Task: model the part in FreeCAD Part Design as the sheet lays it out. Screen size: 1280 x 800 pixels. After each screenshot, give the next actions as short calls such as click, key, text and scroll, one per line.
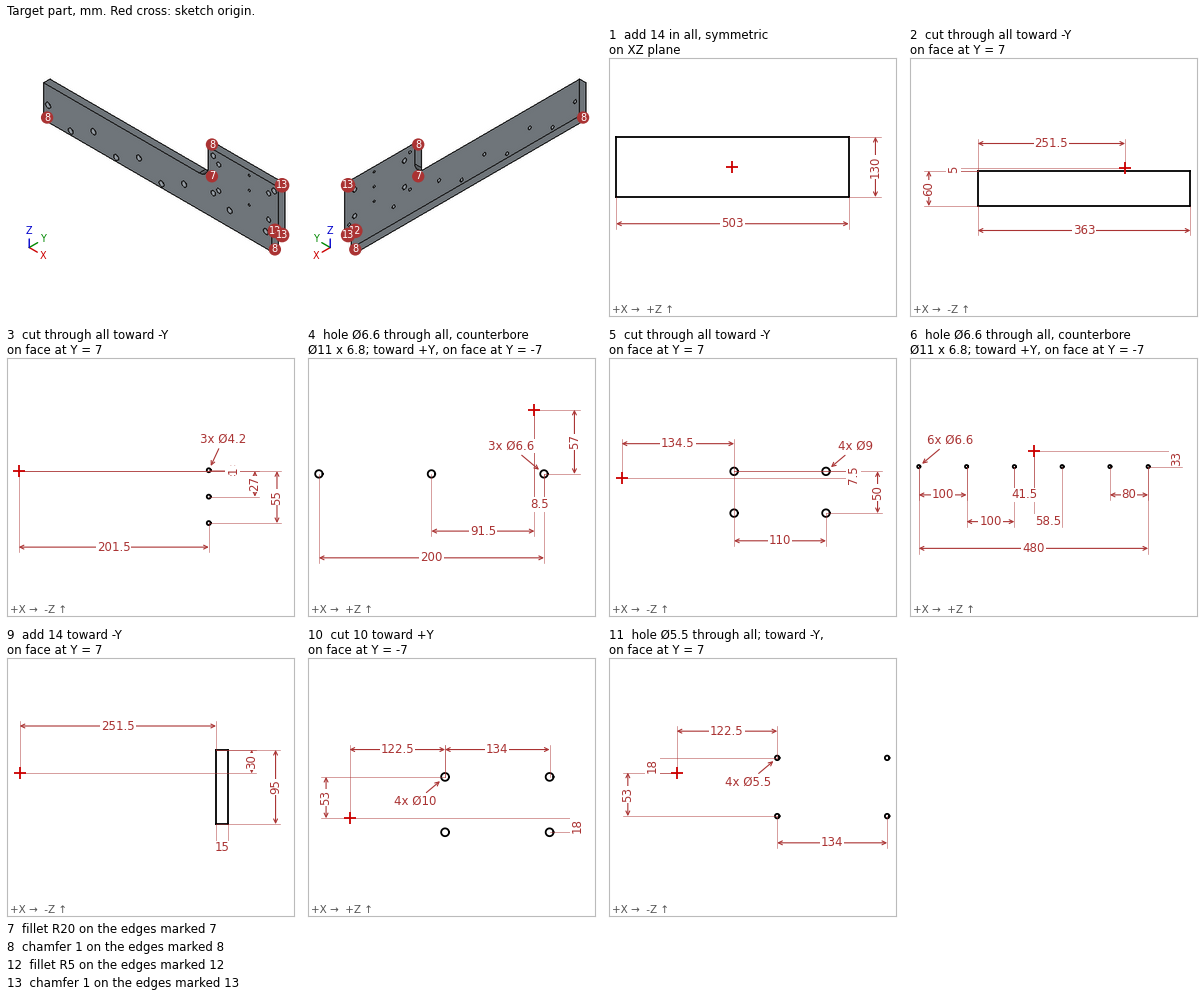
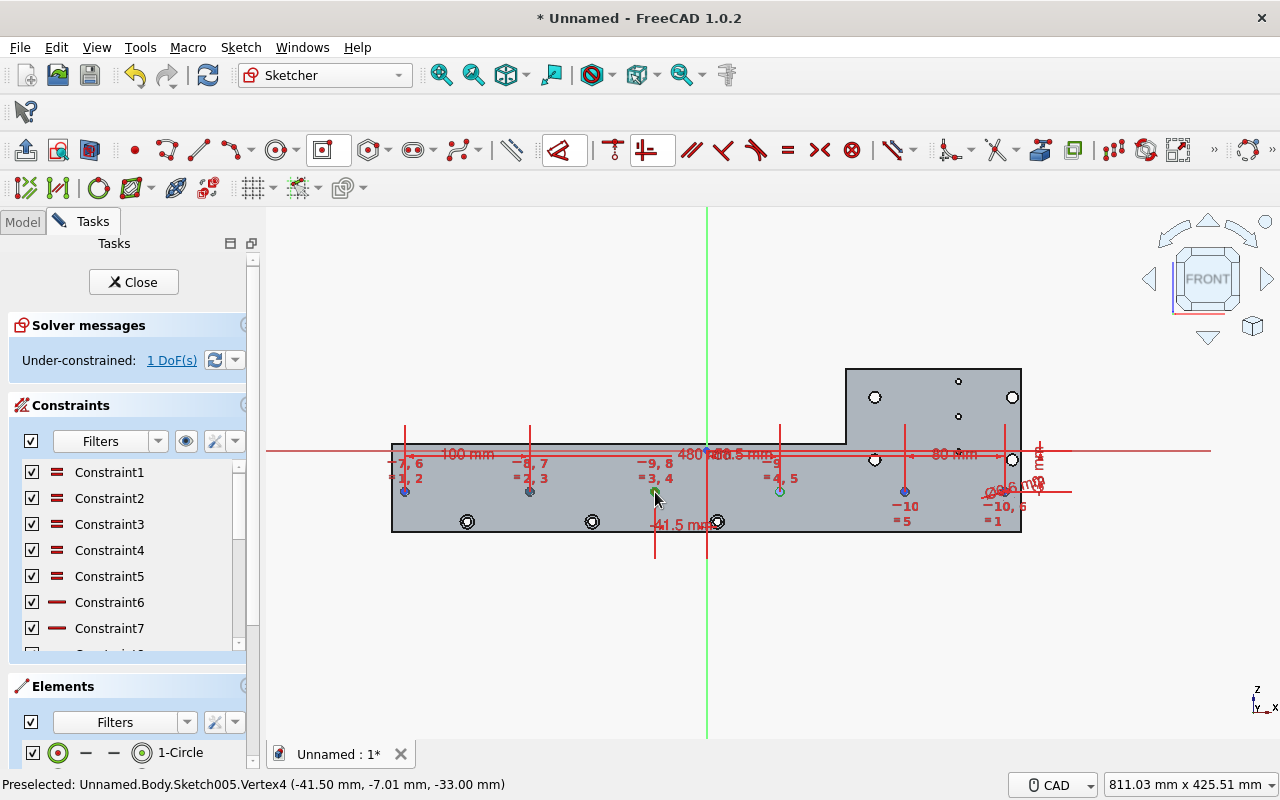
click(582, 150)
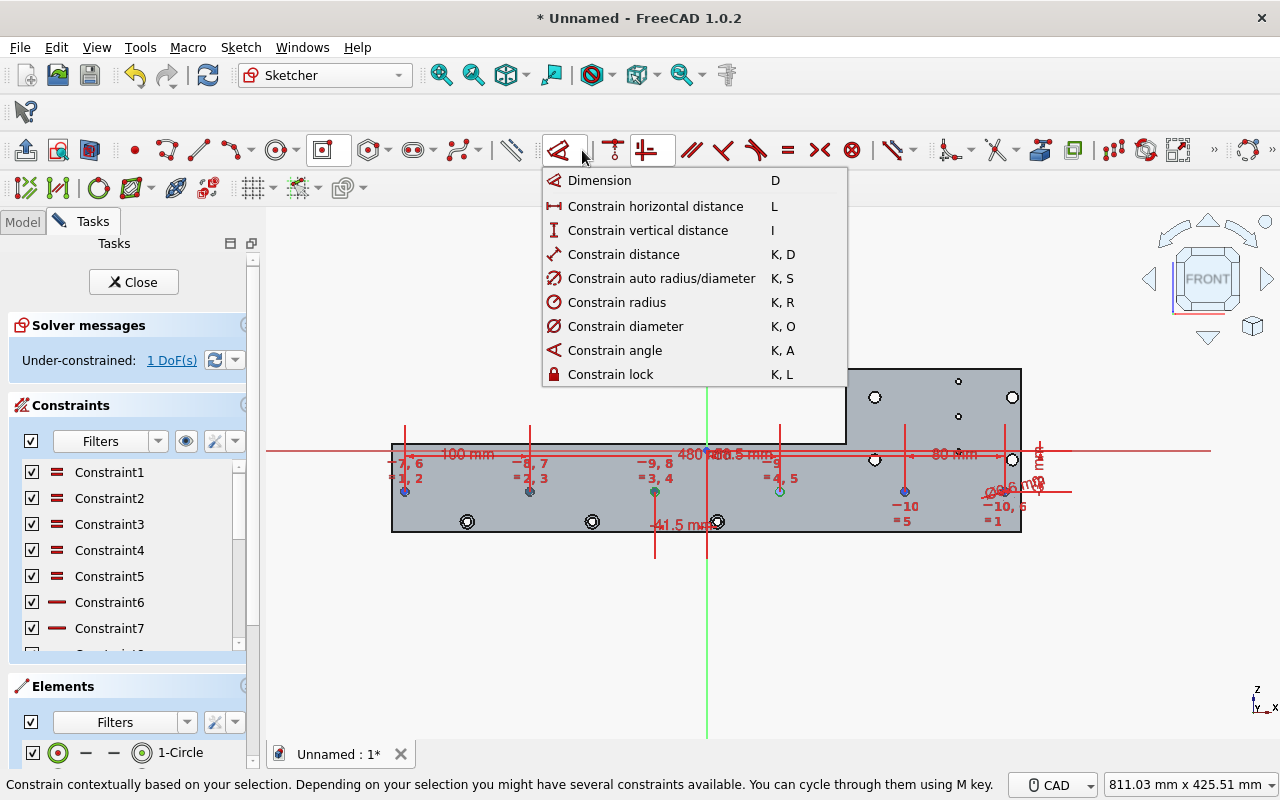
click(695, 206)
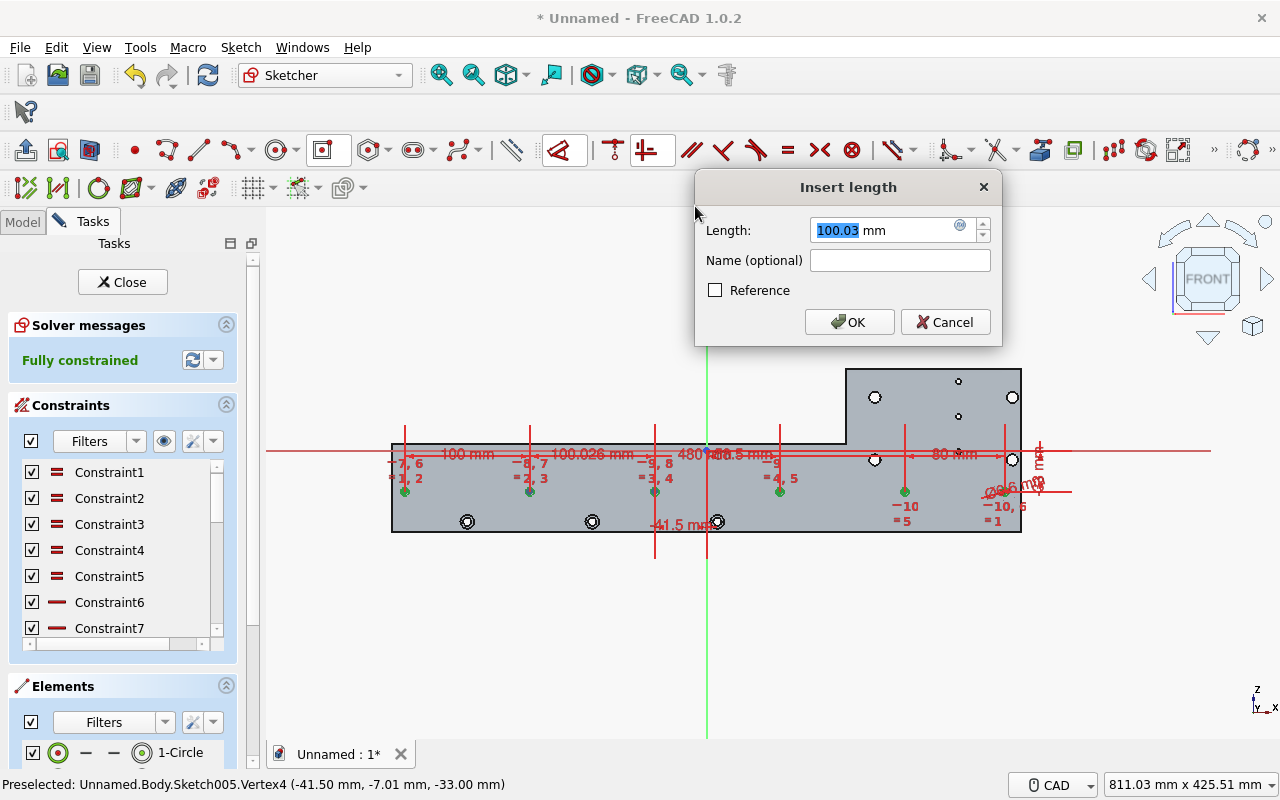
text(100)
key(Return)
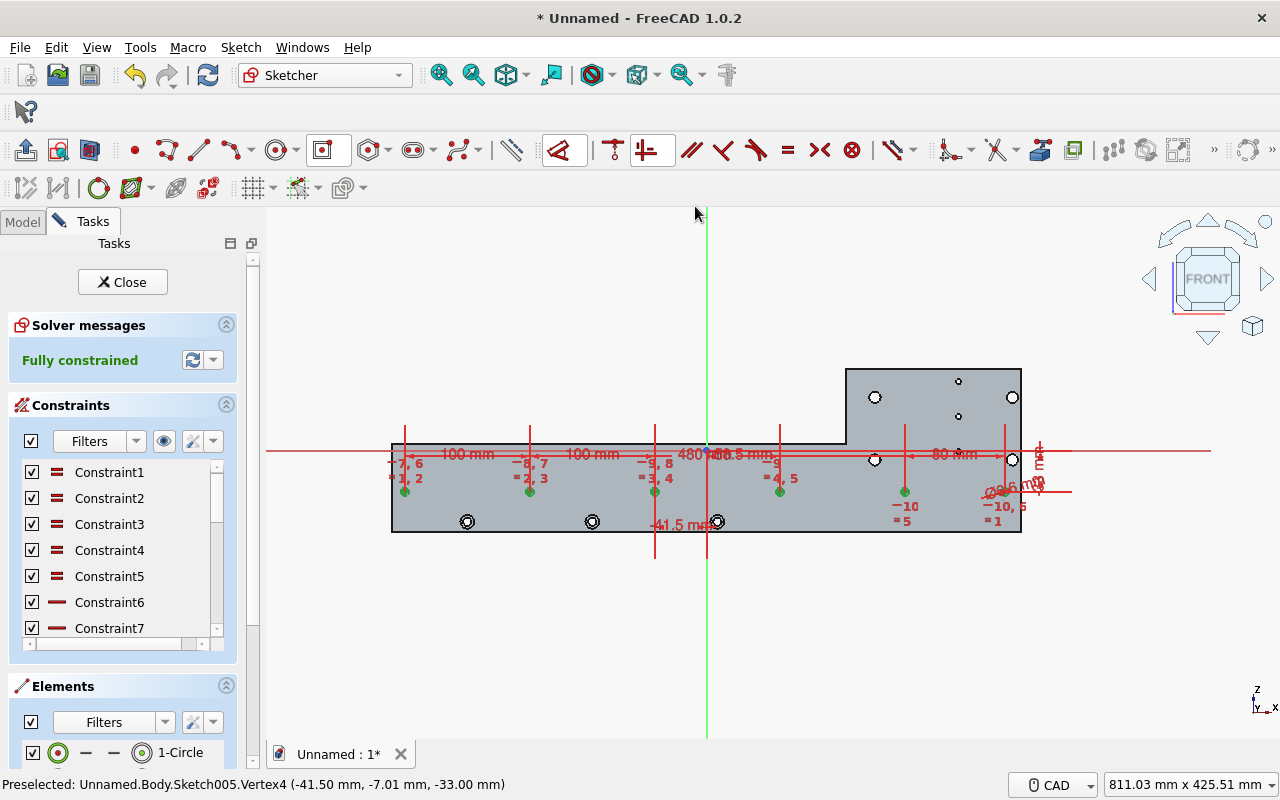
click(123, 282)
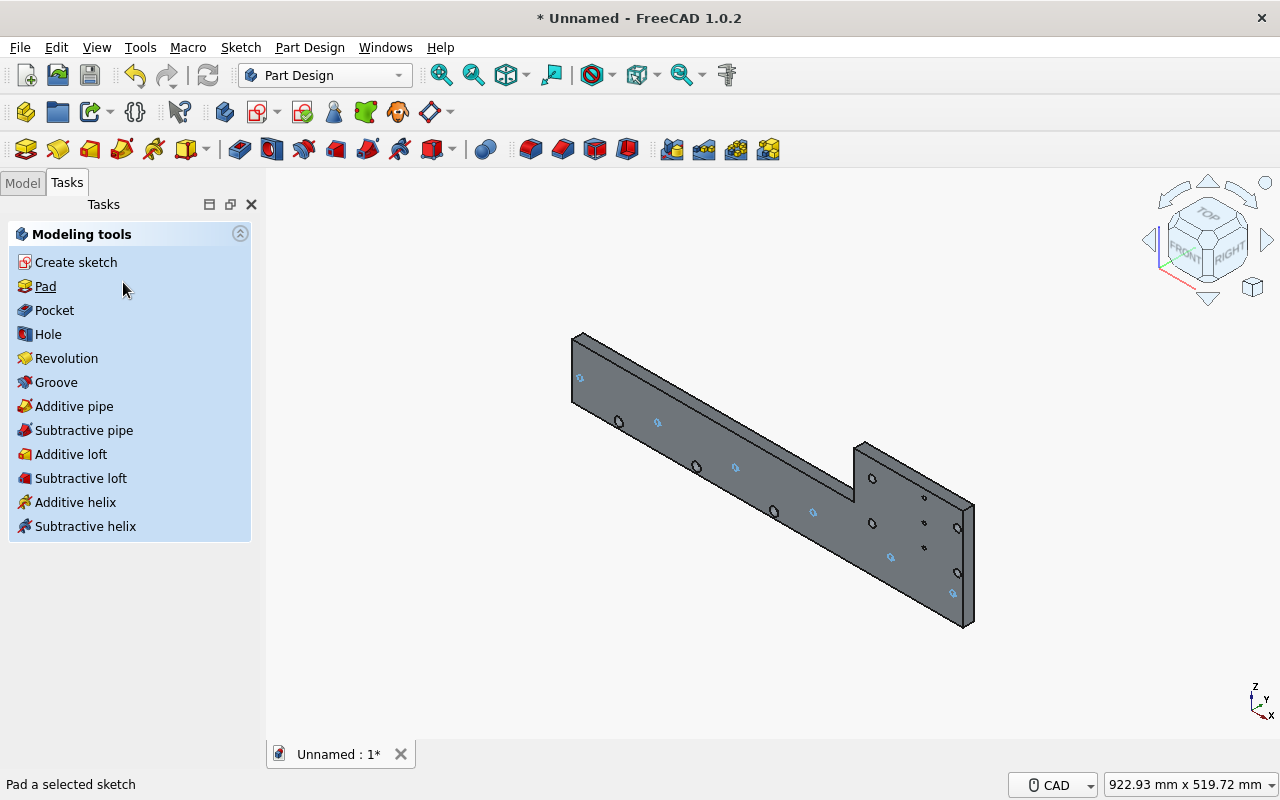
click(272, 150)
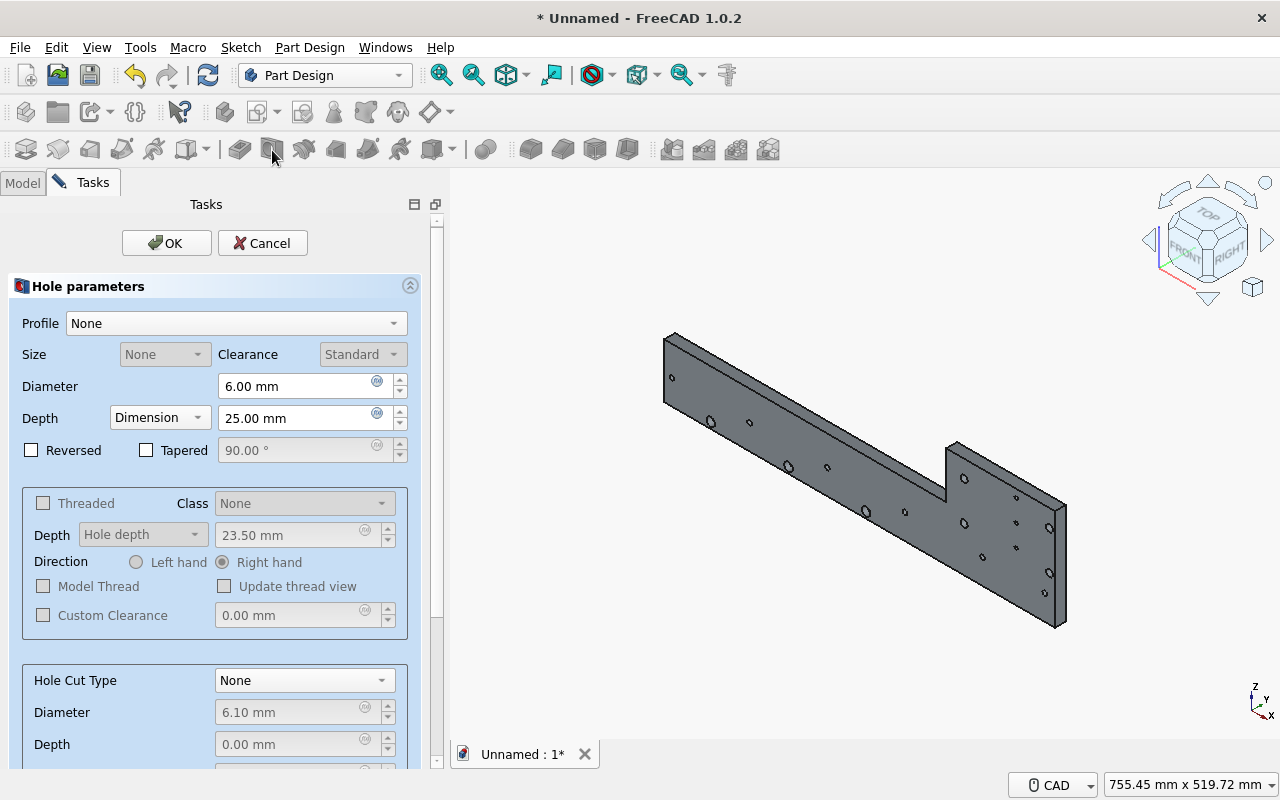
triple_click(305, 386)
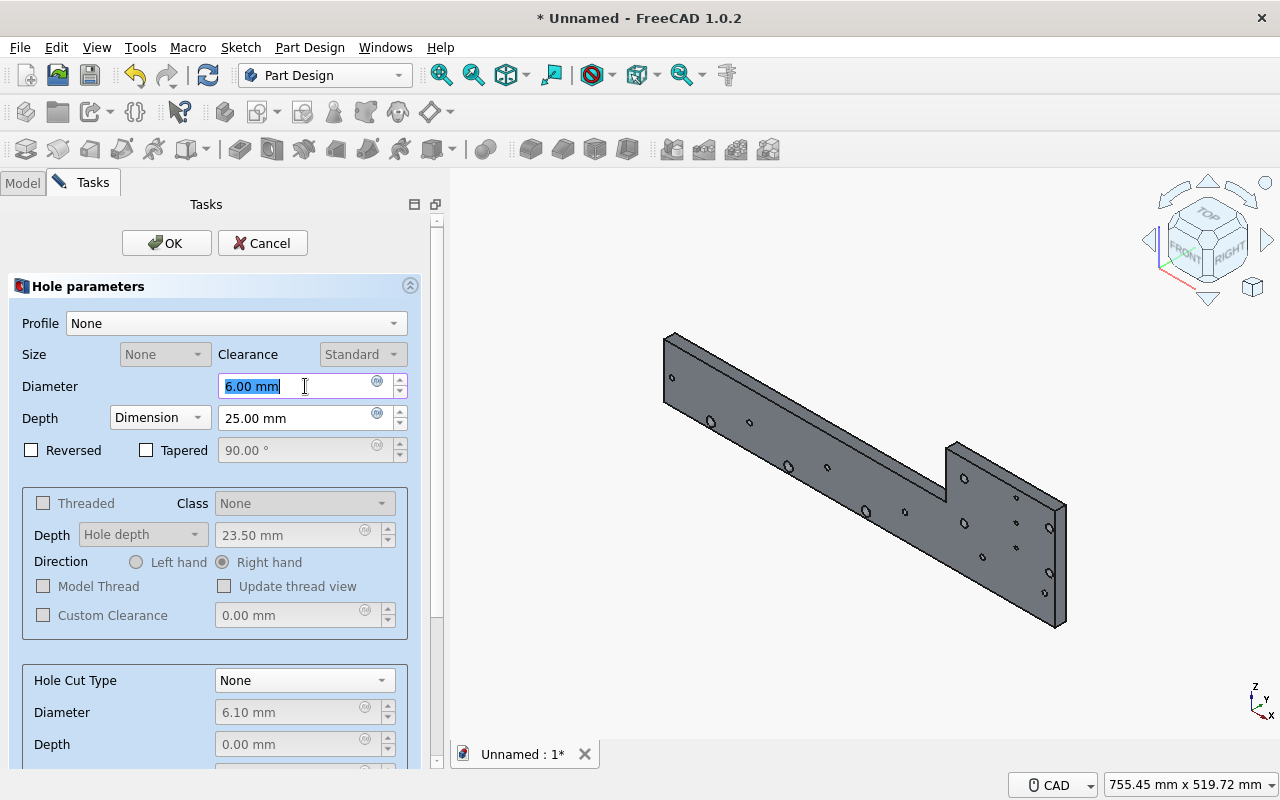
text(6.6)
key(Tab)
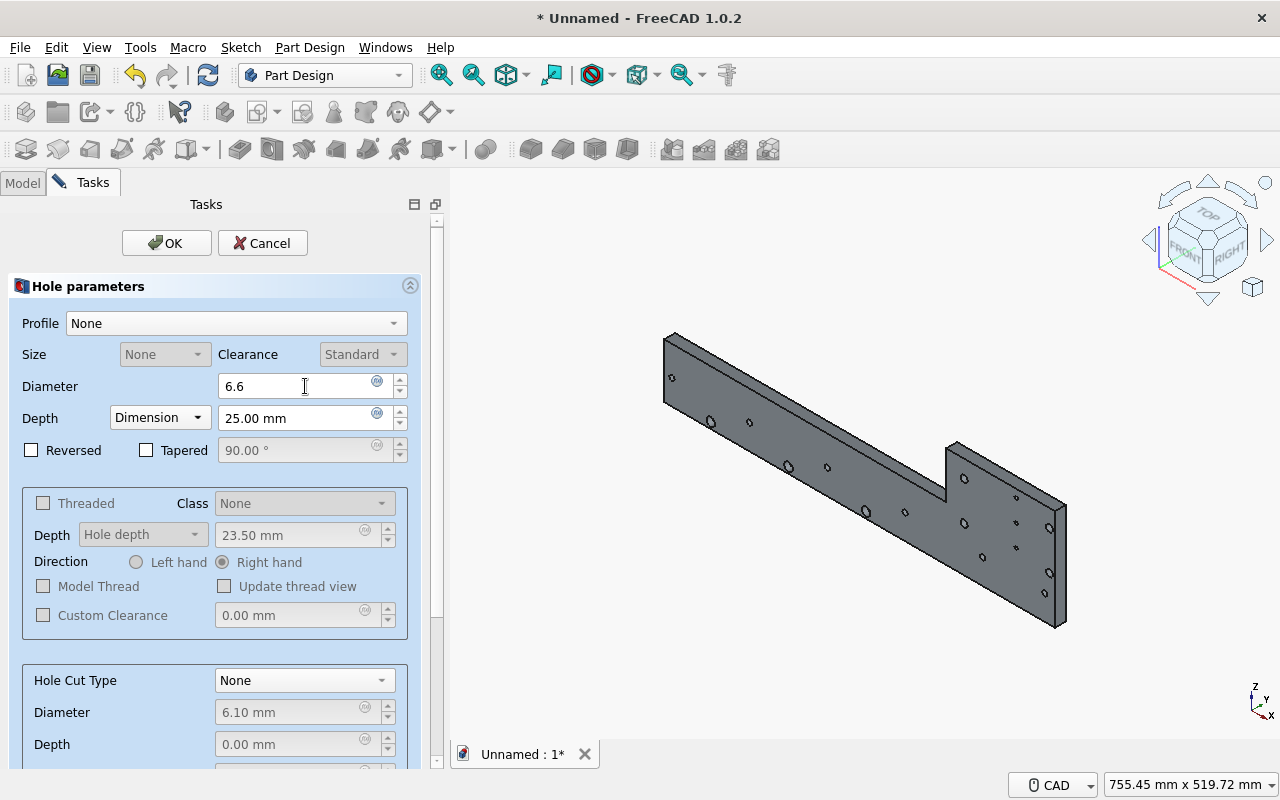
click(161, 418)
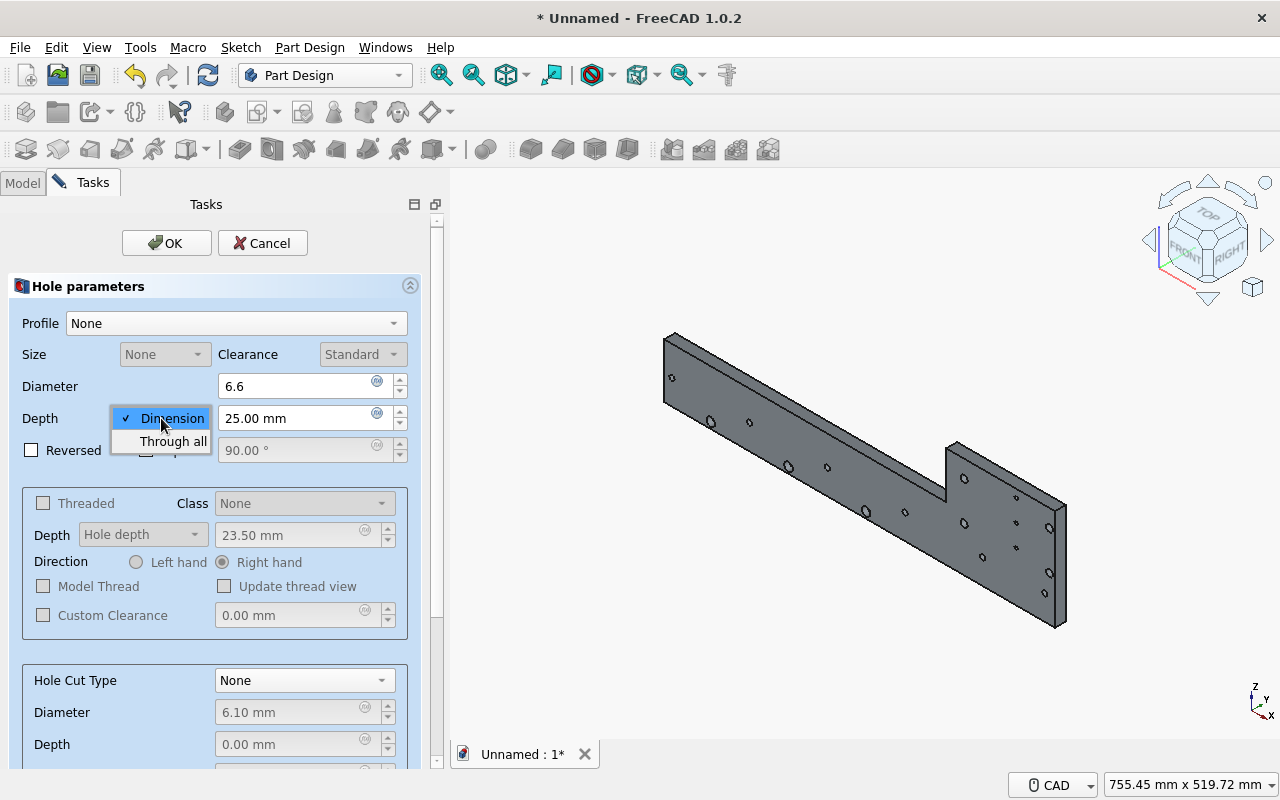
click(160, 442)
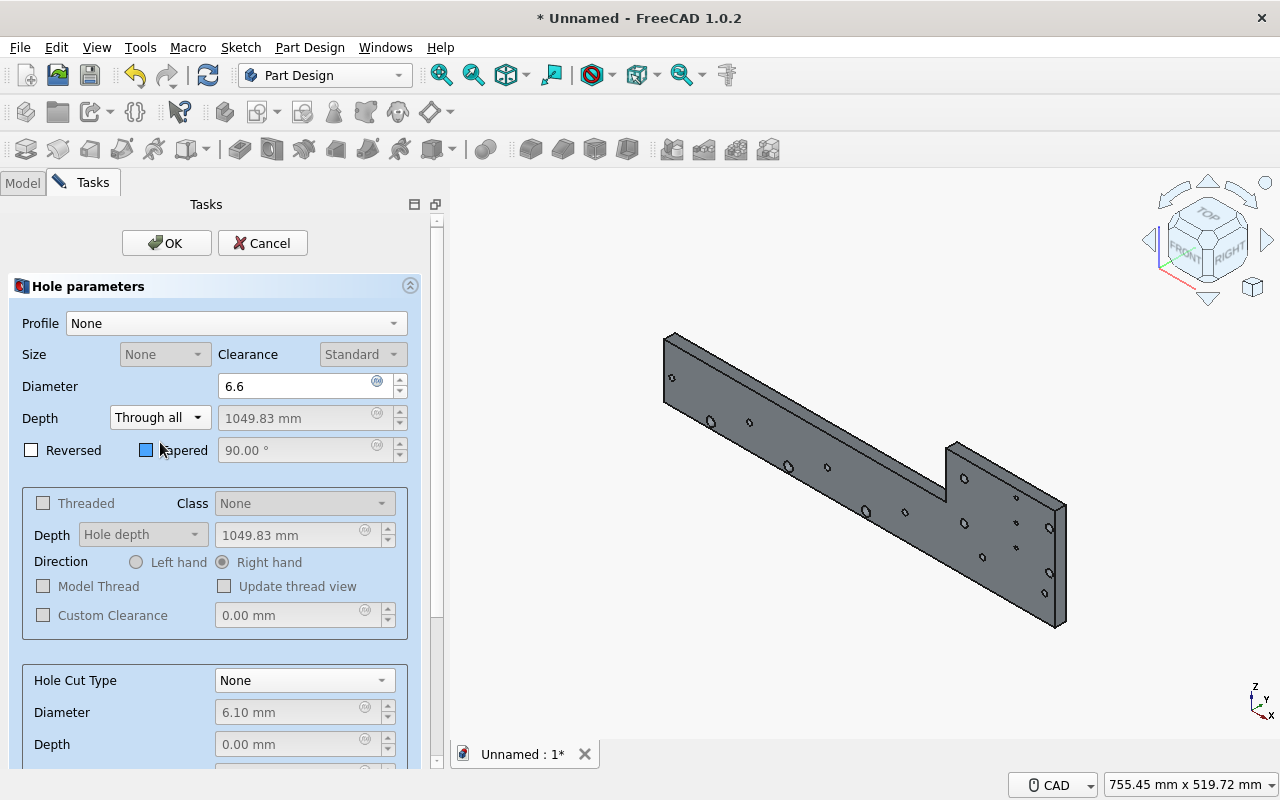
click(306, 680)